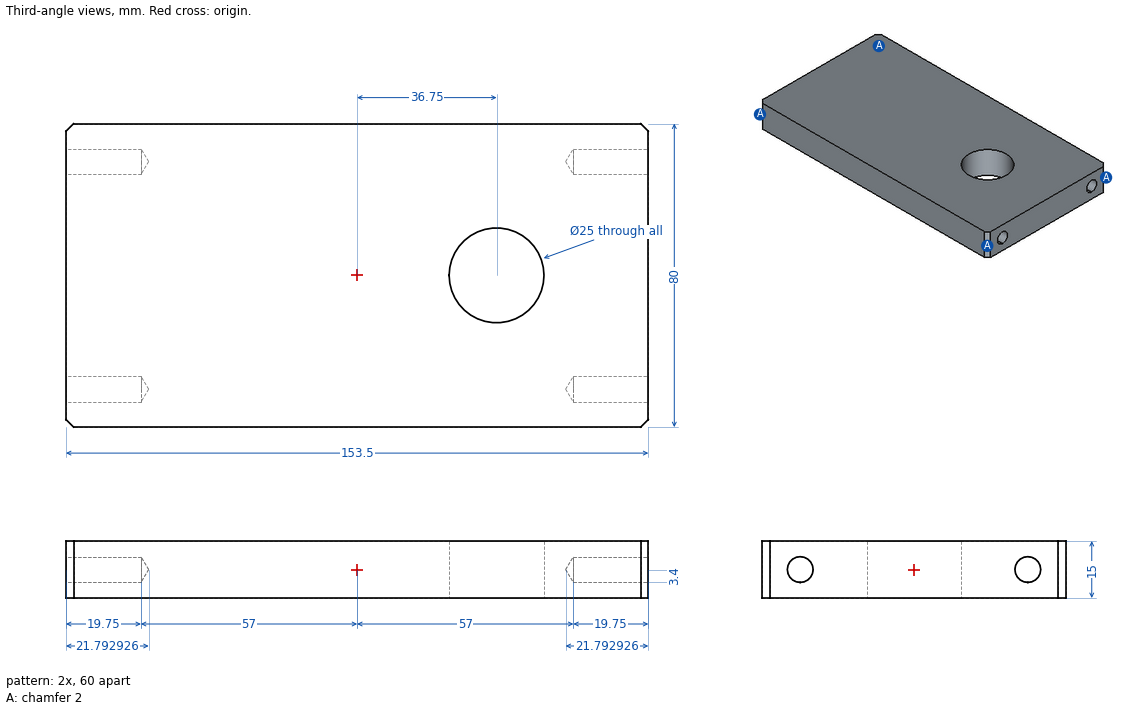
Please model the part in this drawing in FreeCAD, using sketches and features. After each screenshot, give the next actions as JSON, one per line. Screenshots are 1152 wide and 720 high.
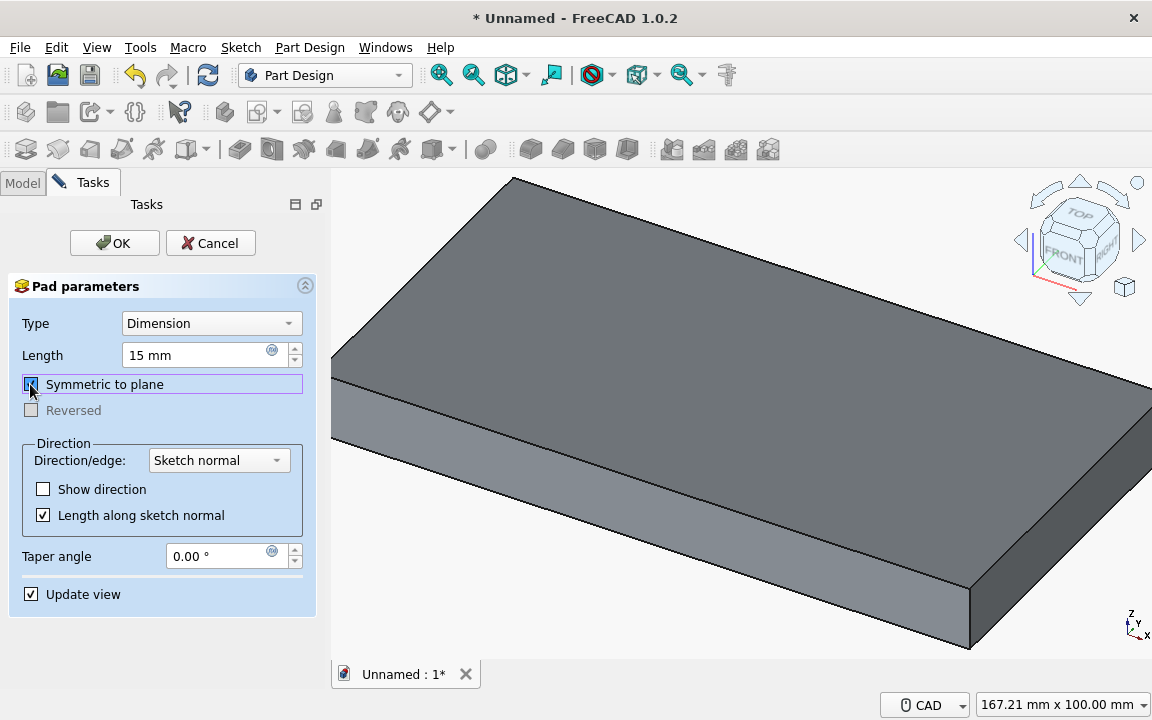
{"action": "left_click", "coordinate": [115, 243]}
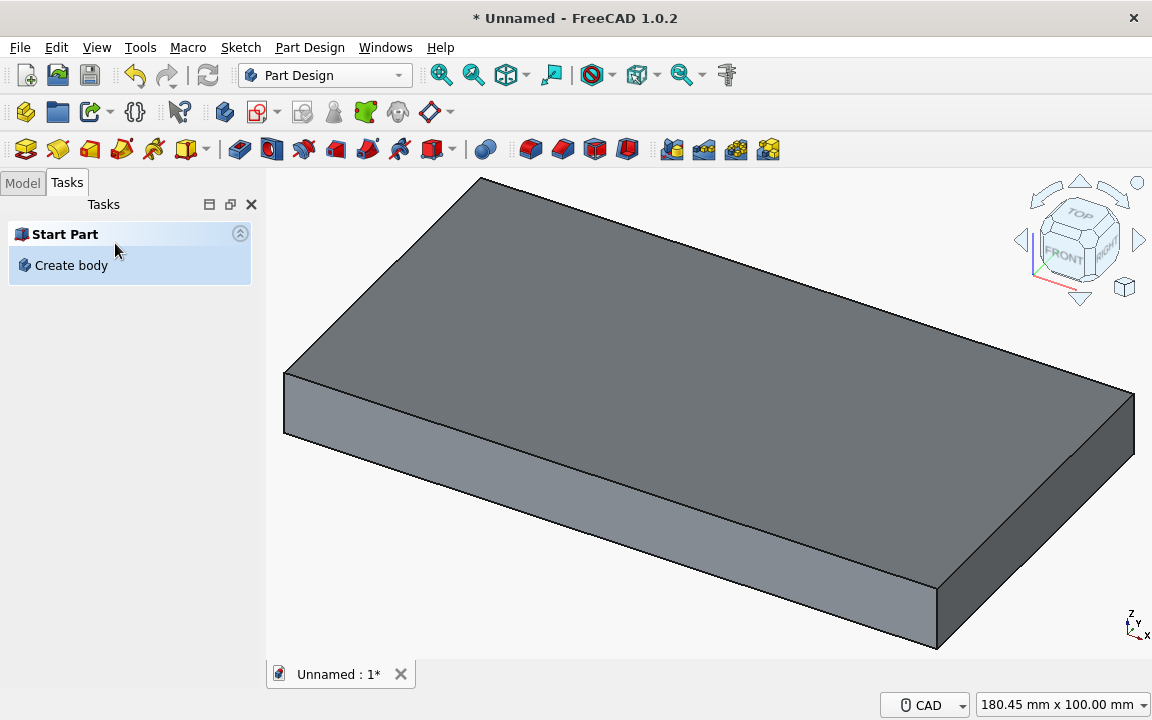
{"action": "left_click", "coordinate": [802, 413]}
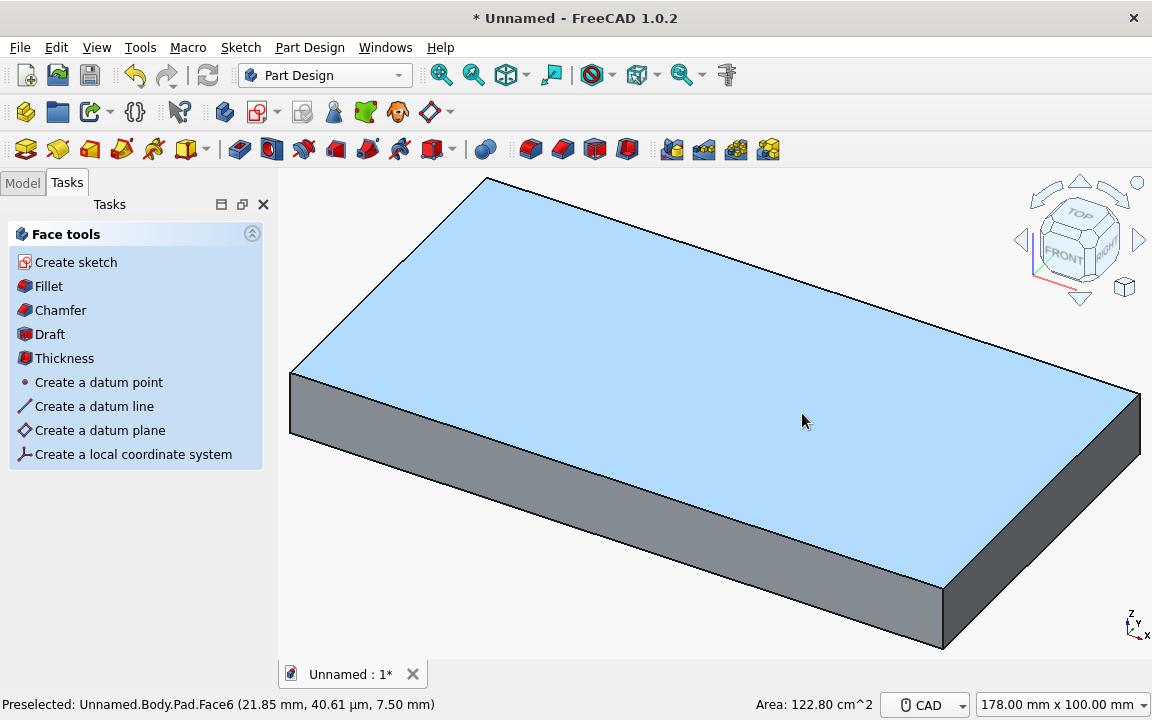
{"action": "left_click", "coordinate": [258, 112]}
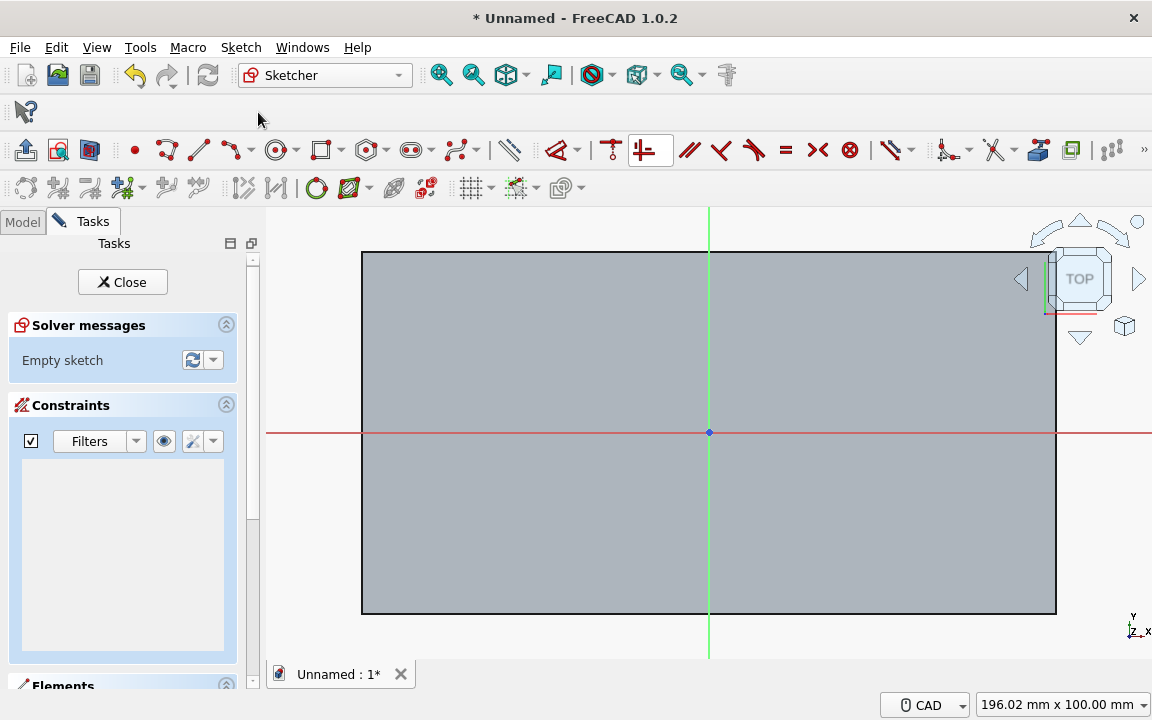
{"action": "scroll", "coordinate": [967, 433], "scroll_direction": "up", "scroll_amount": 4}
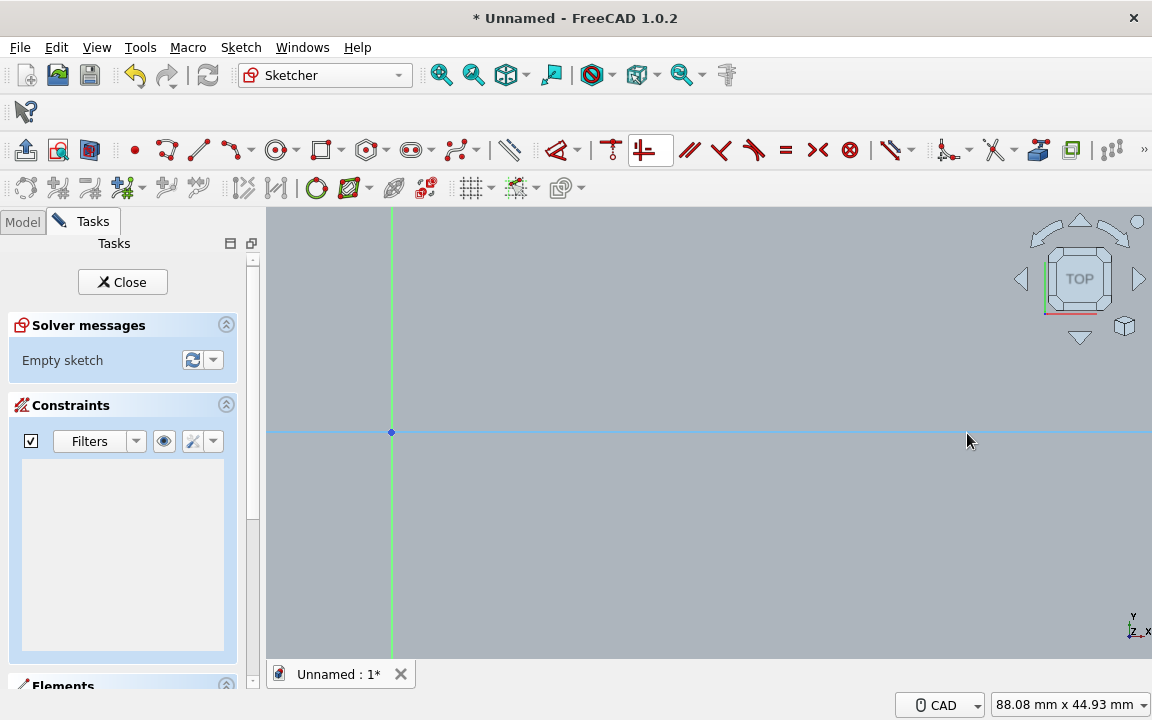
{"action": "left_click", "coordinate": [276, 150]}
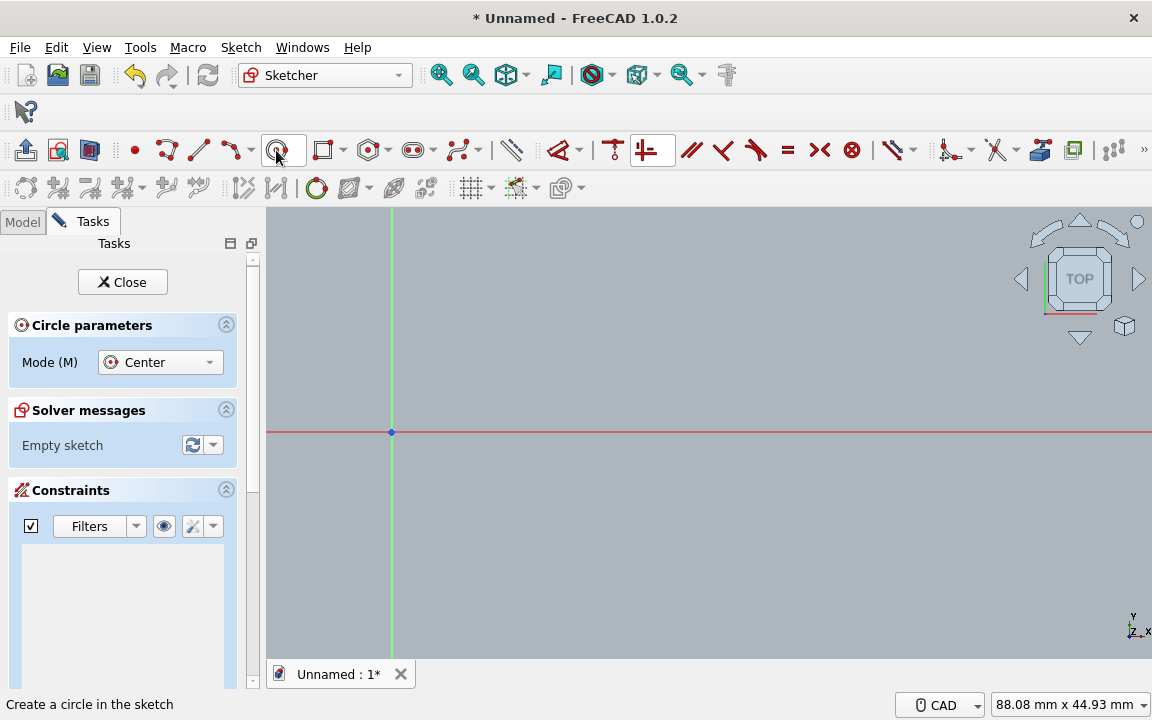
{"action": "left_click", "coordinate": [762, 432]}
{"action": "mouse_move", "coordinate": [850, 343]}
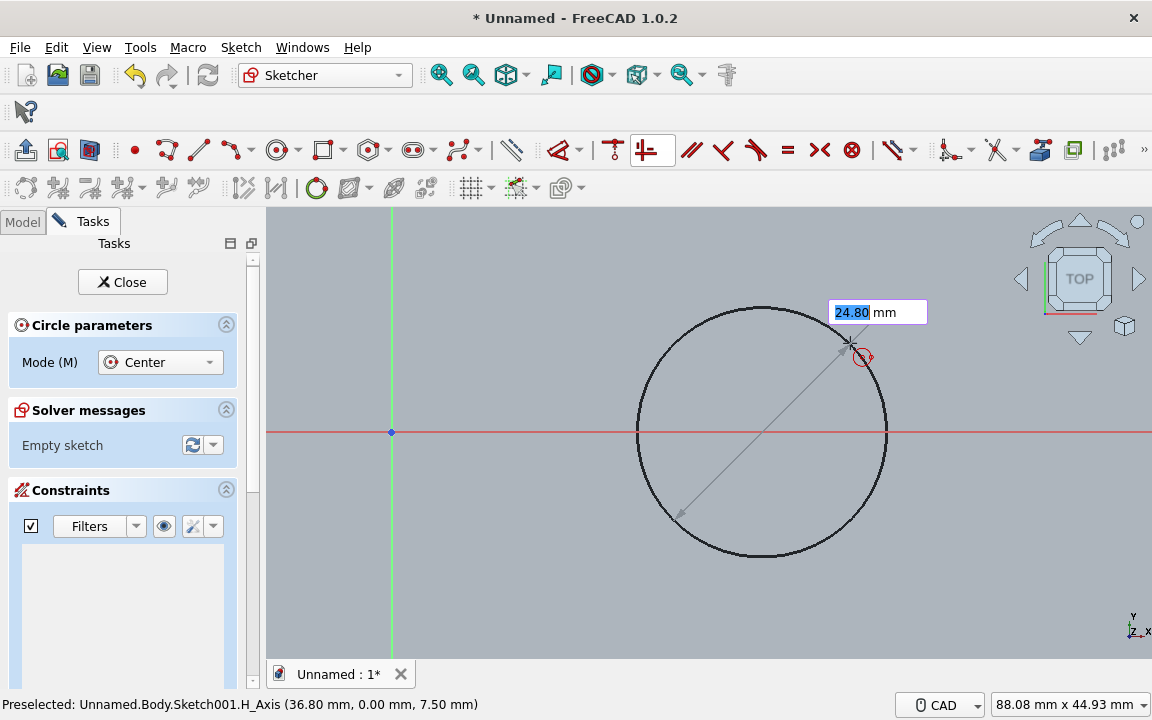
{"action": "type", "text": "25"}
{"action": "key", "text": "Return"}
{"action": "key", "text": "Escape"}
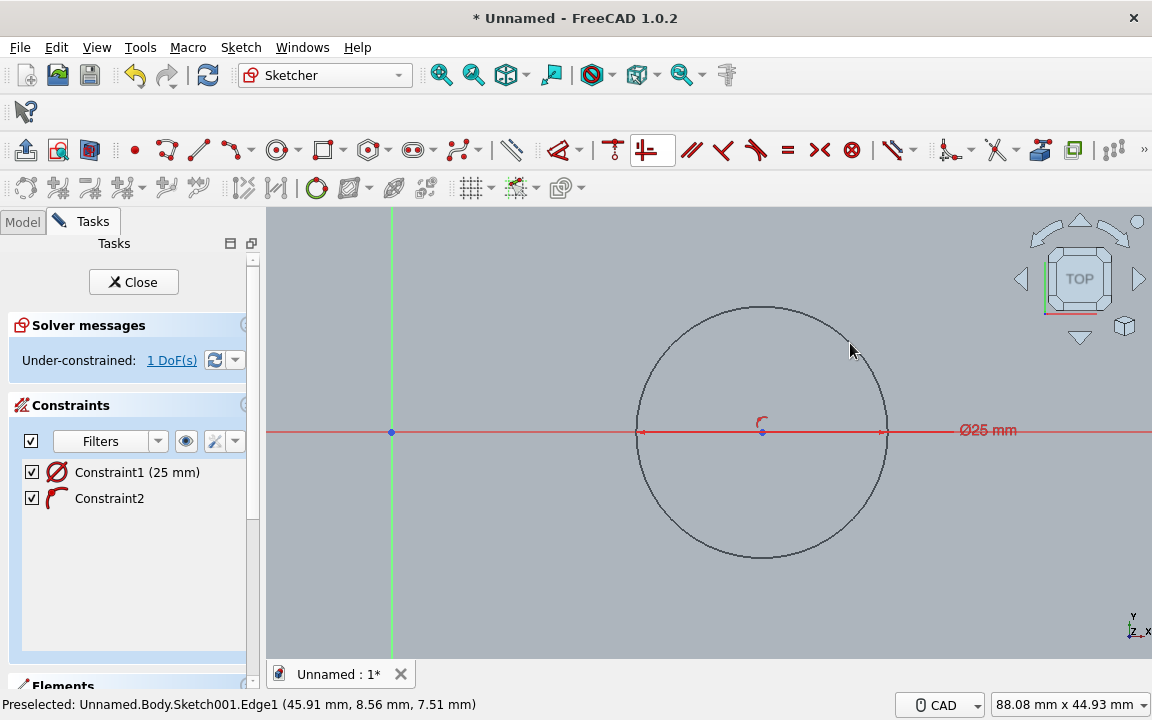
{"action": "key", "text": "d"}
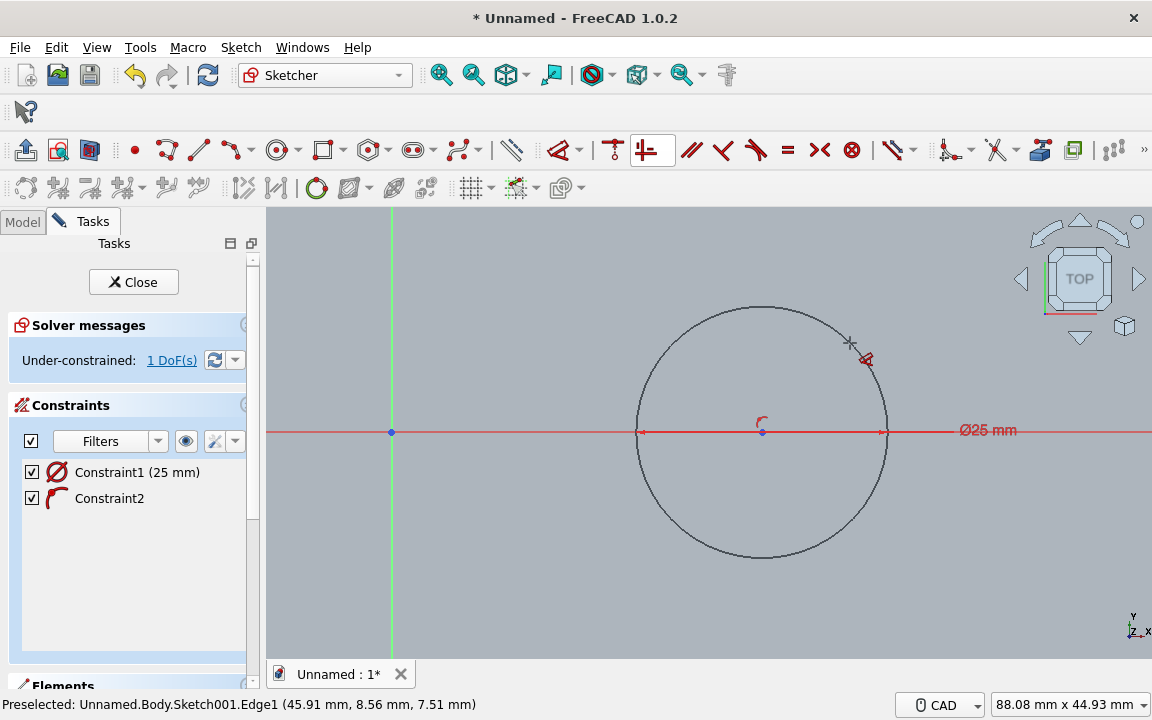
{"action": "left_click", "coordinate": [762, 432]}
{"action": "left_click", "coordinate": [577, 466]}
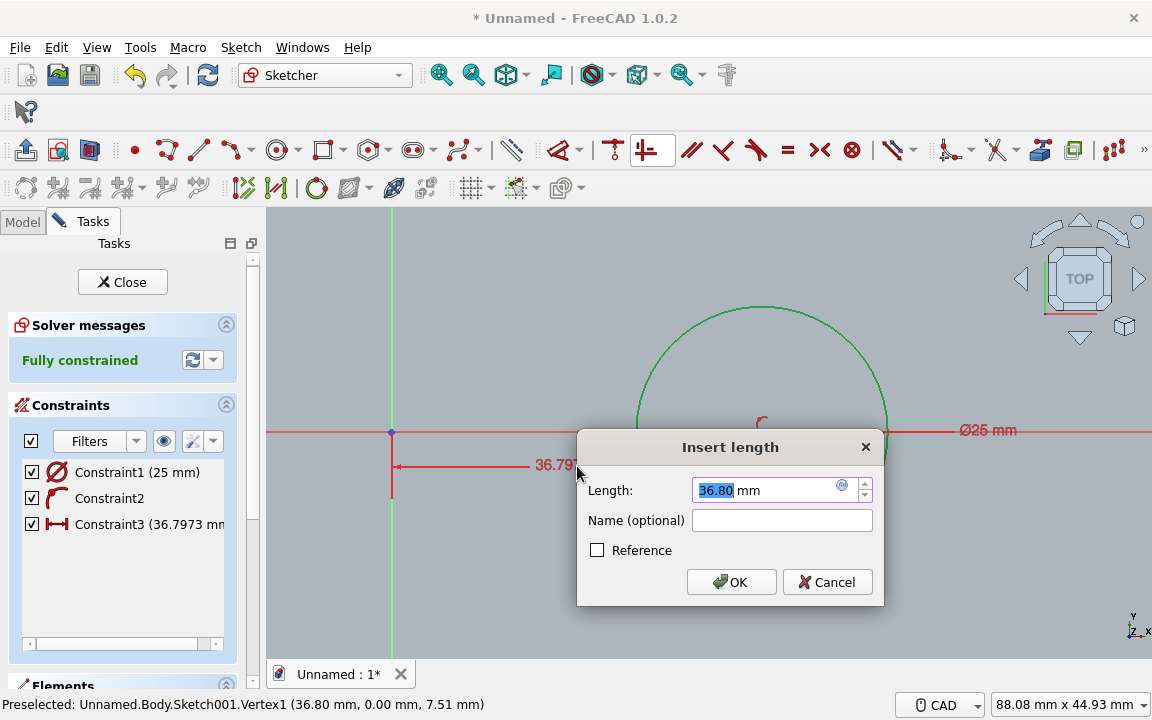
{"action": "type", "text": "36.75"}
{"action": "key", "text": "Return"}
{"action": "key", "text": "Escape"}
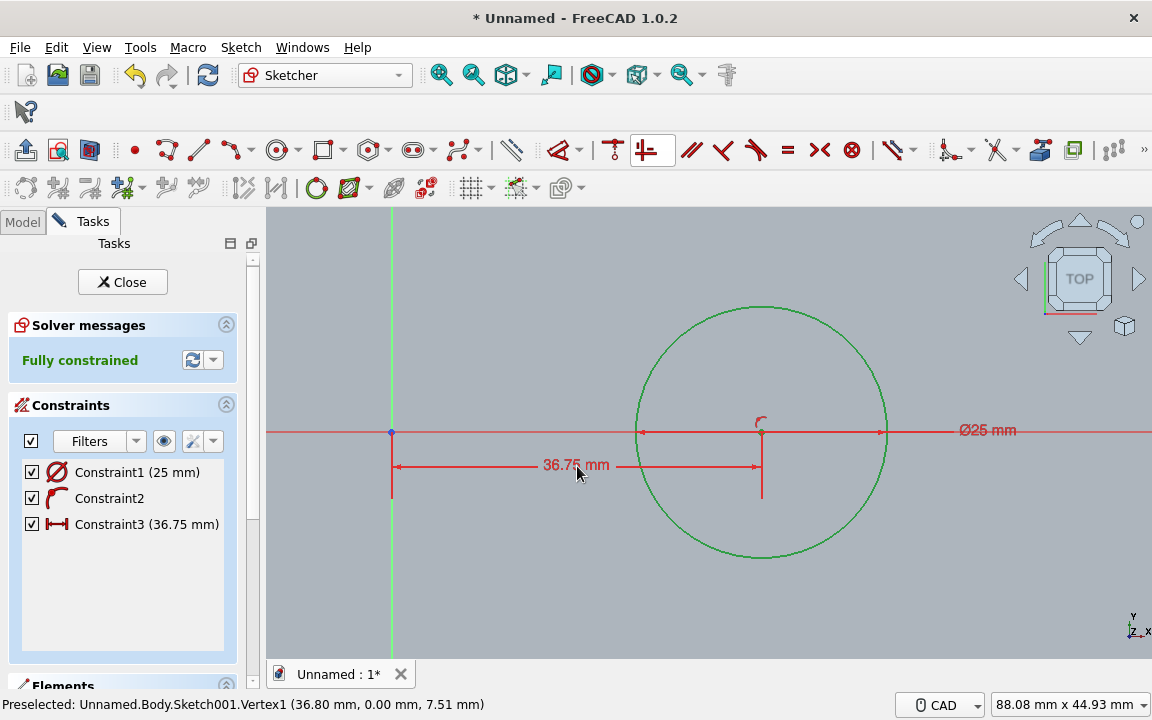
{"action": "left_click", "coordinate": [123, 282]}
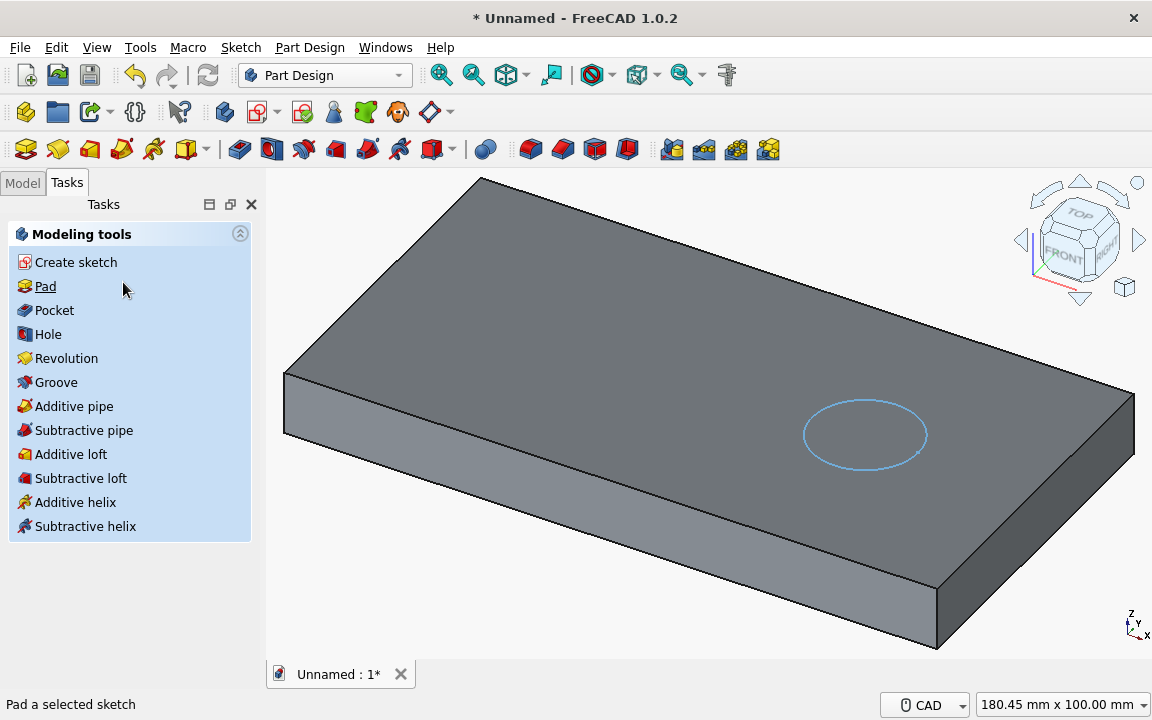
{"action": "left_click", "coordinate": [272, 150]}